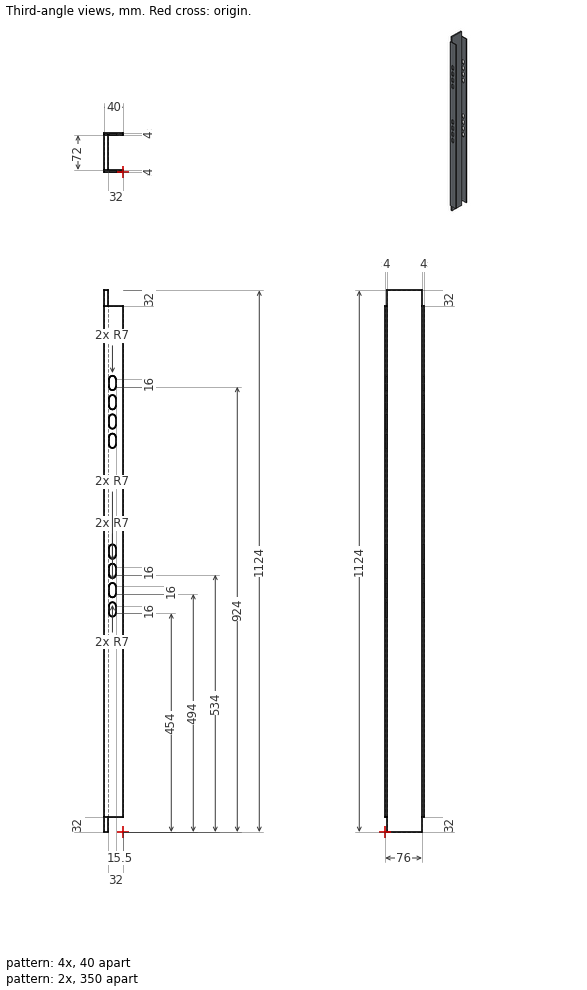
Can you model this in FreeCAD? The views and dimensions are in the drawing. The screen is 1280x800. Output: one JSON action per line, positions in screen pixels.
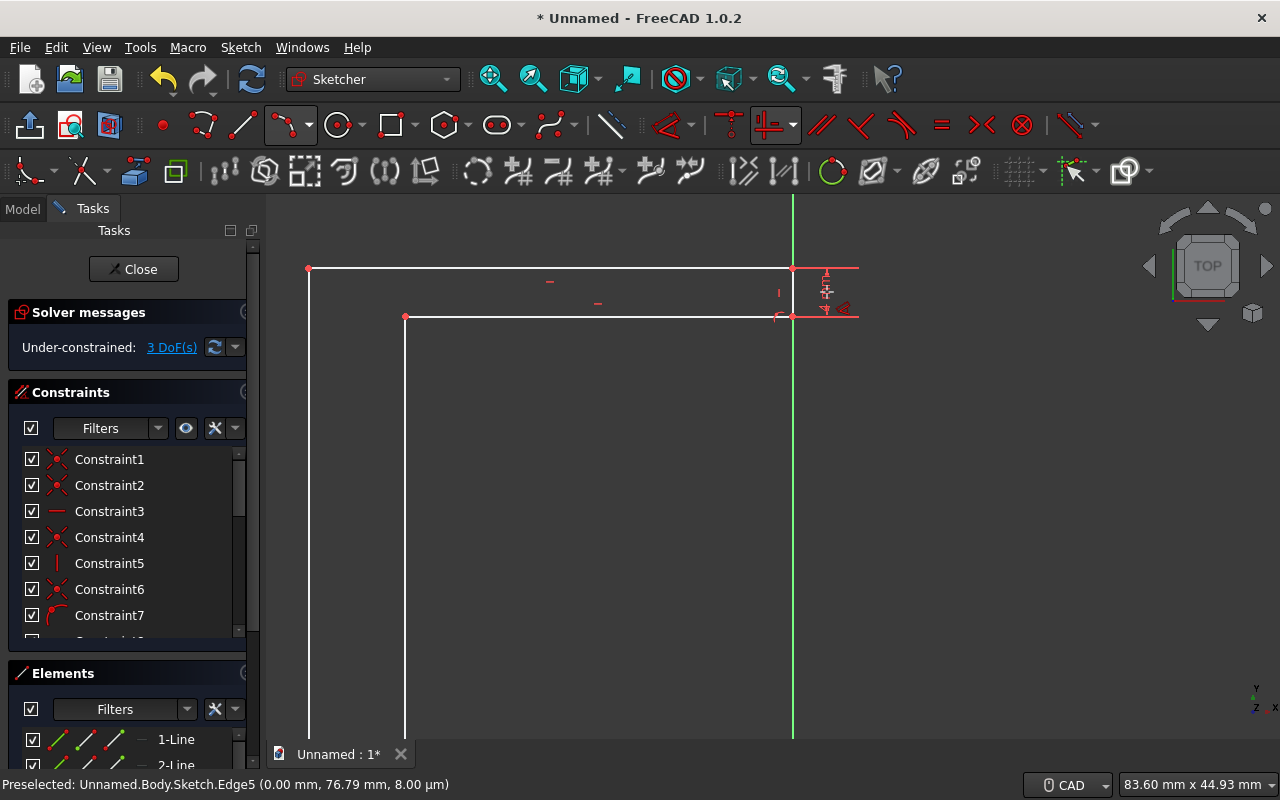
{"action": "scroll", "coordinate": [794, 302], "scroll_direction": "down", "scroll_amount": 5}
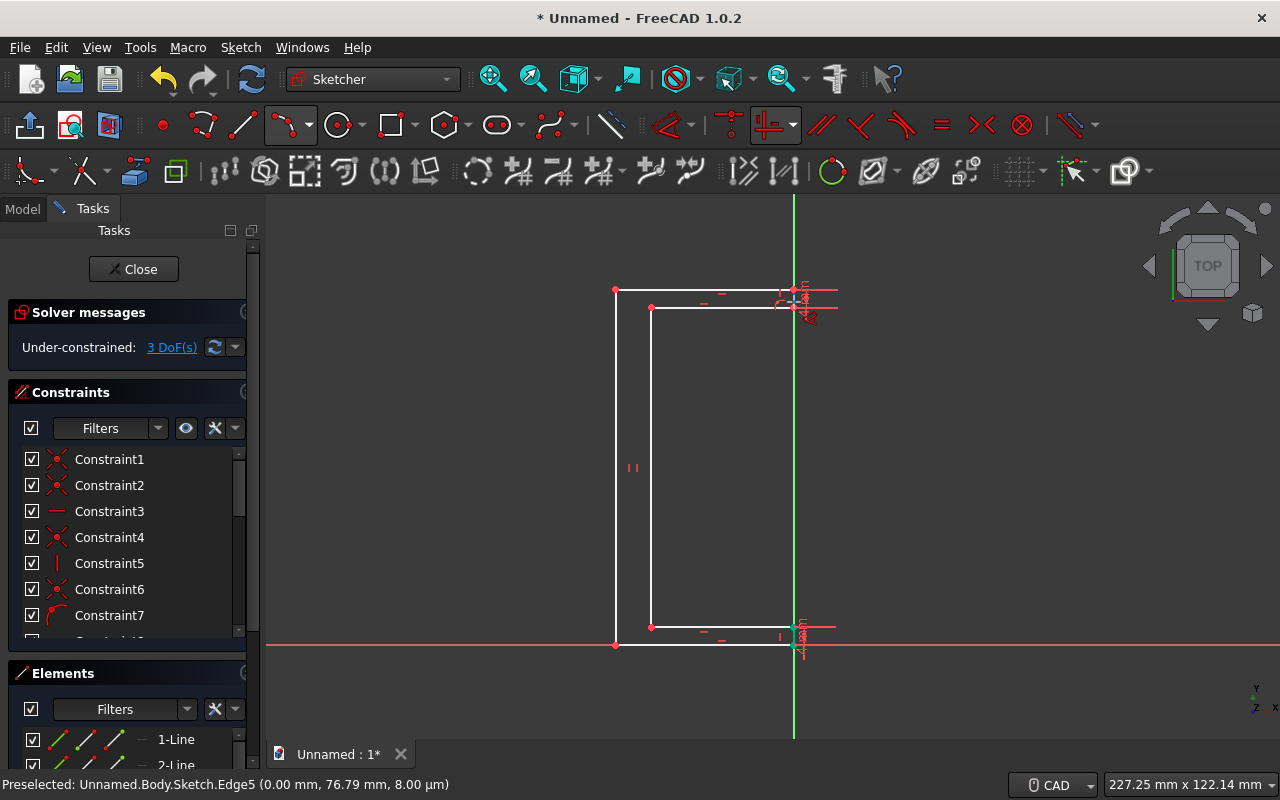
{"action": "left_click", "coordinate": [751, 627]}
{"action": "left_click", "coordinate": [723, 661]}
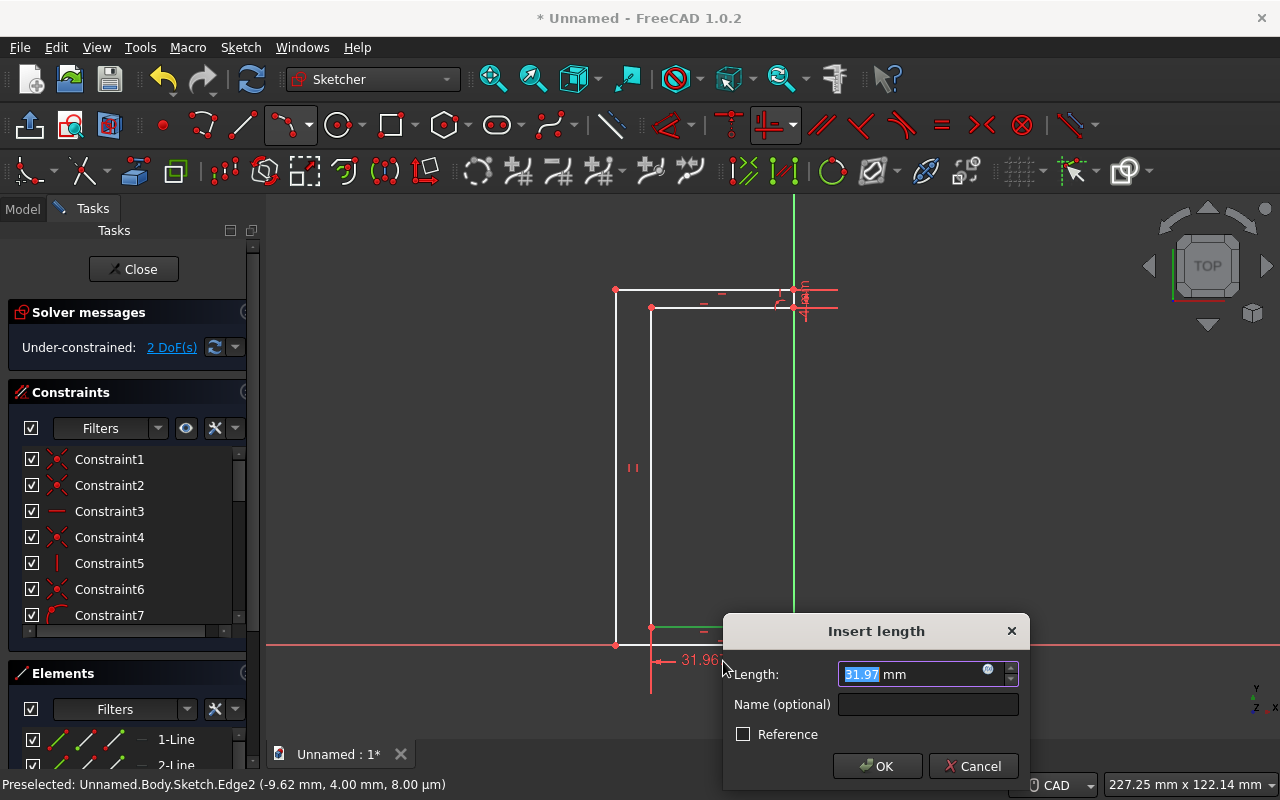
{"action": "type", "text": "32"}
{"action": "key", "text": "Return"}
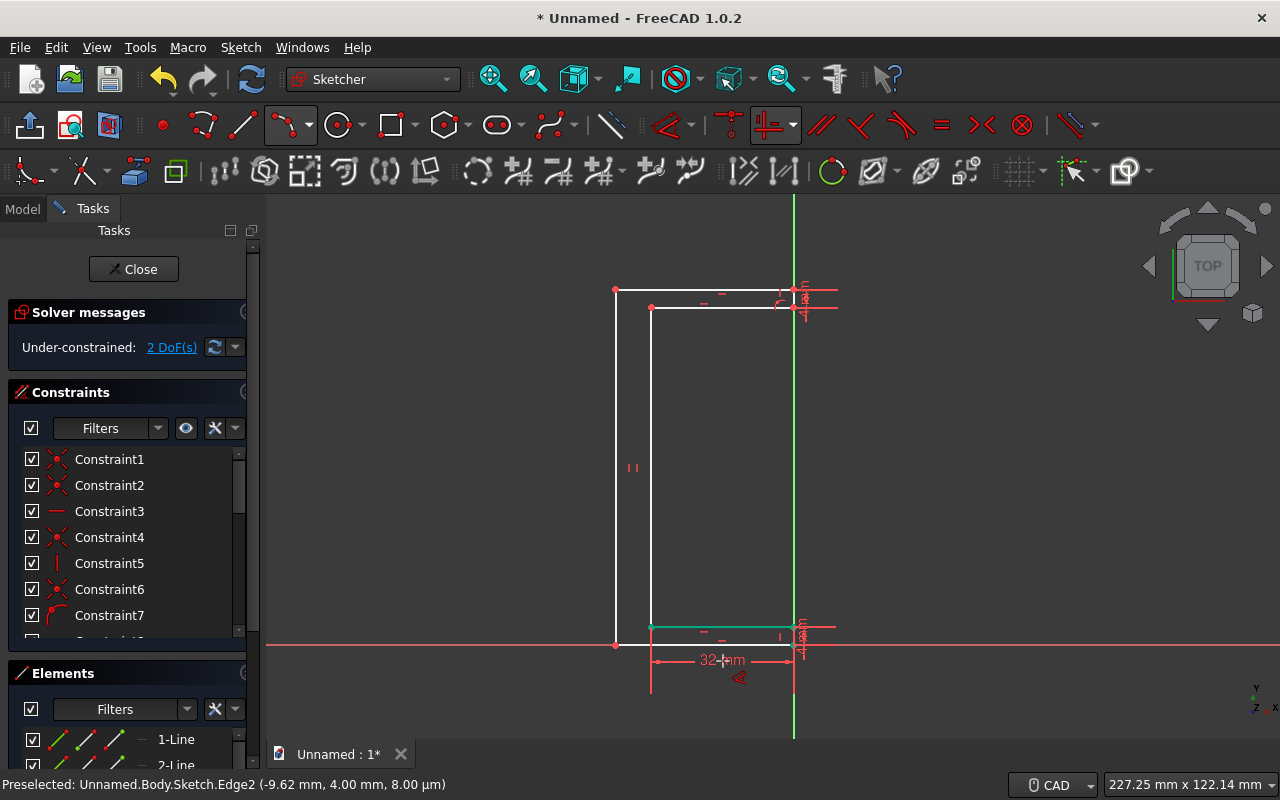
{"action": "left_click", "coordinate": [651, 531]}
{"action": "left_click", "coordinate": [685, 467]}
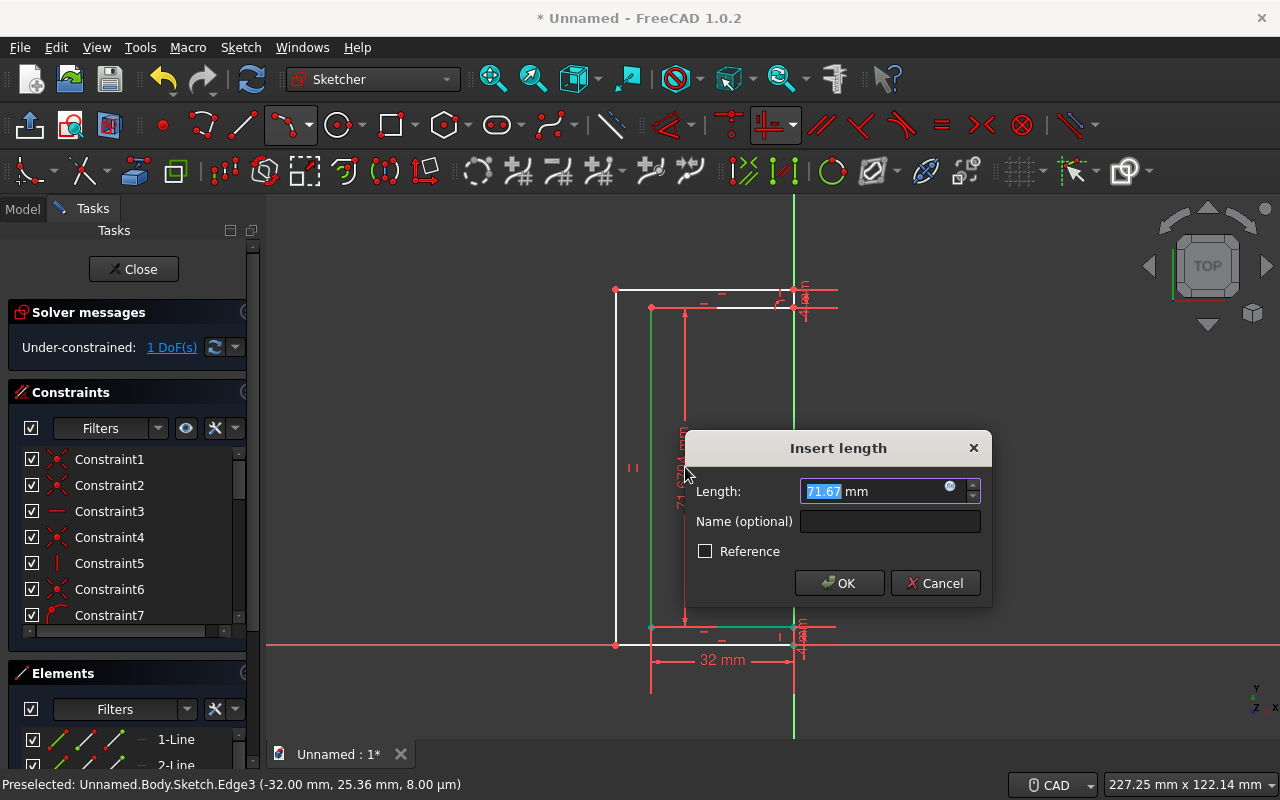
{"action": "type", "text": "72"}
{"action": "key", "text": "Return"}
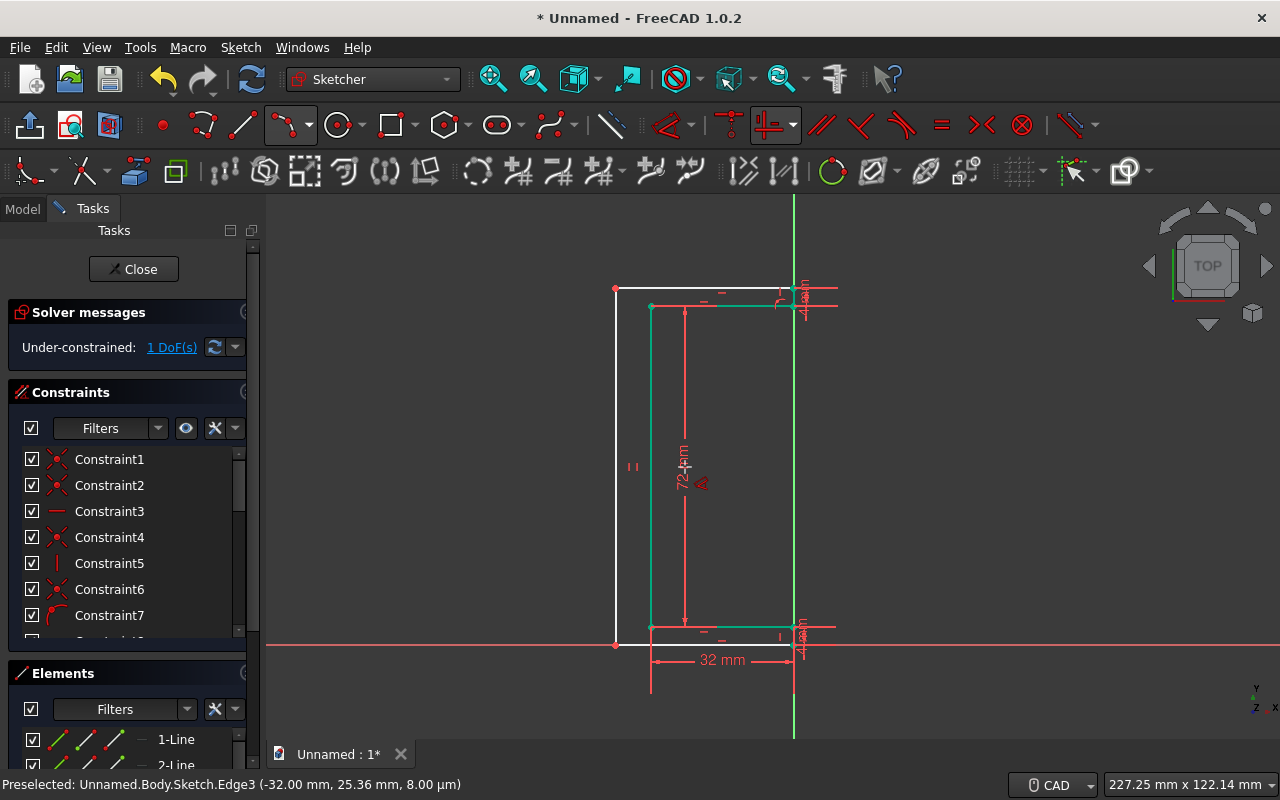
{"action": "left_click", "coordinate": [740, 288]}
{"action": "left_click", "coordinate": [705, 254]}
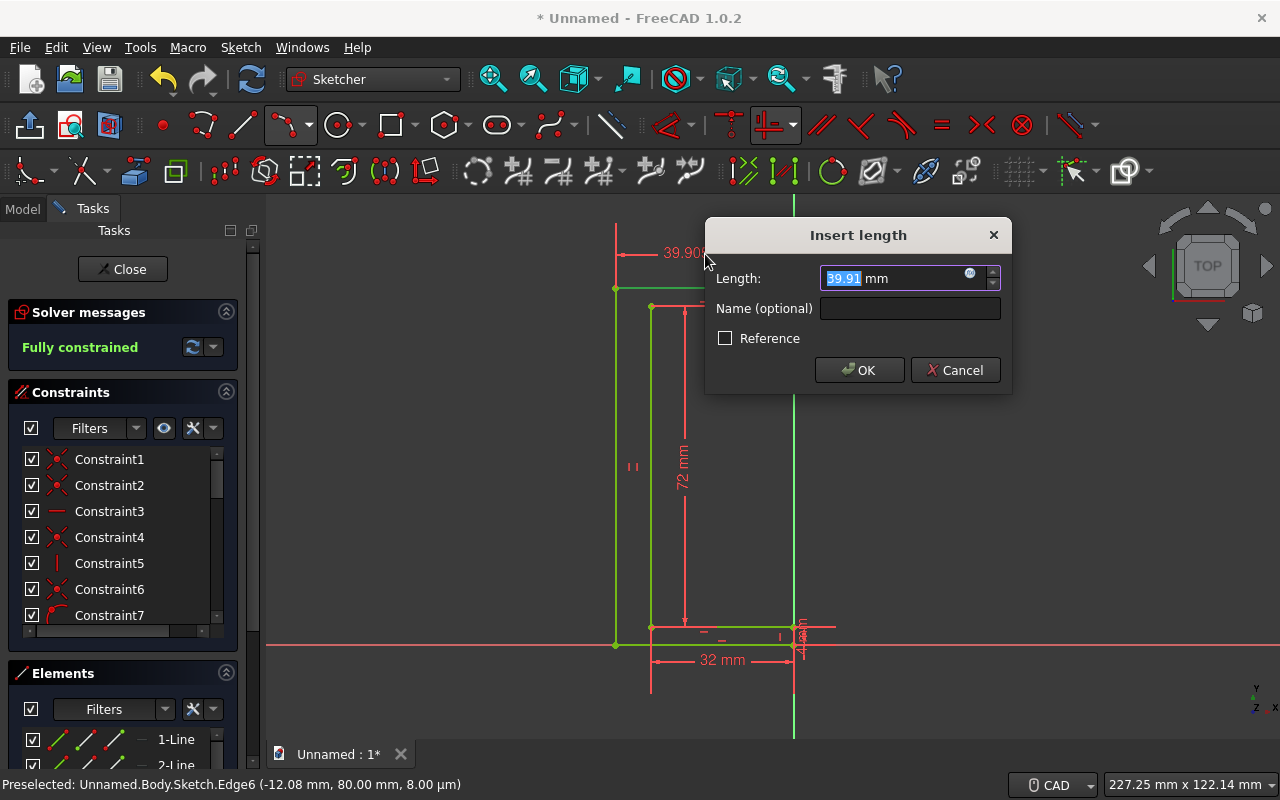
{"action": "type", "text": "40"}
{"action": "key", "text": "Return"}
{"action": "key", "text": "Escape"}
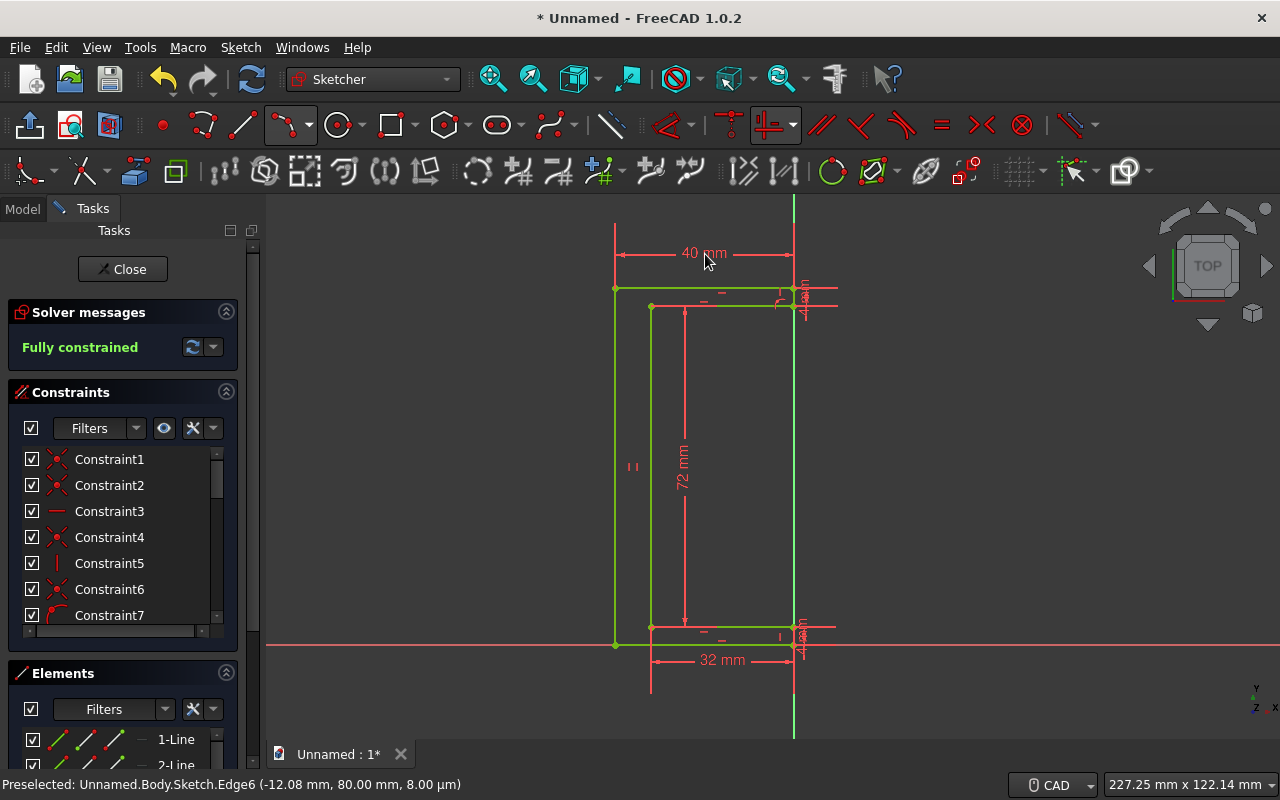
{"action": "left_click", "coordinate": [123, 269]}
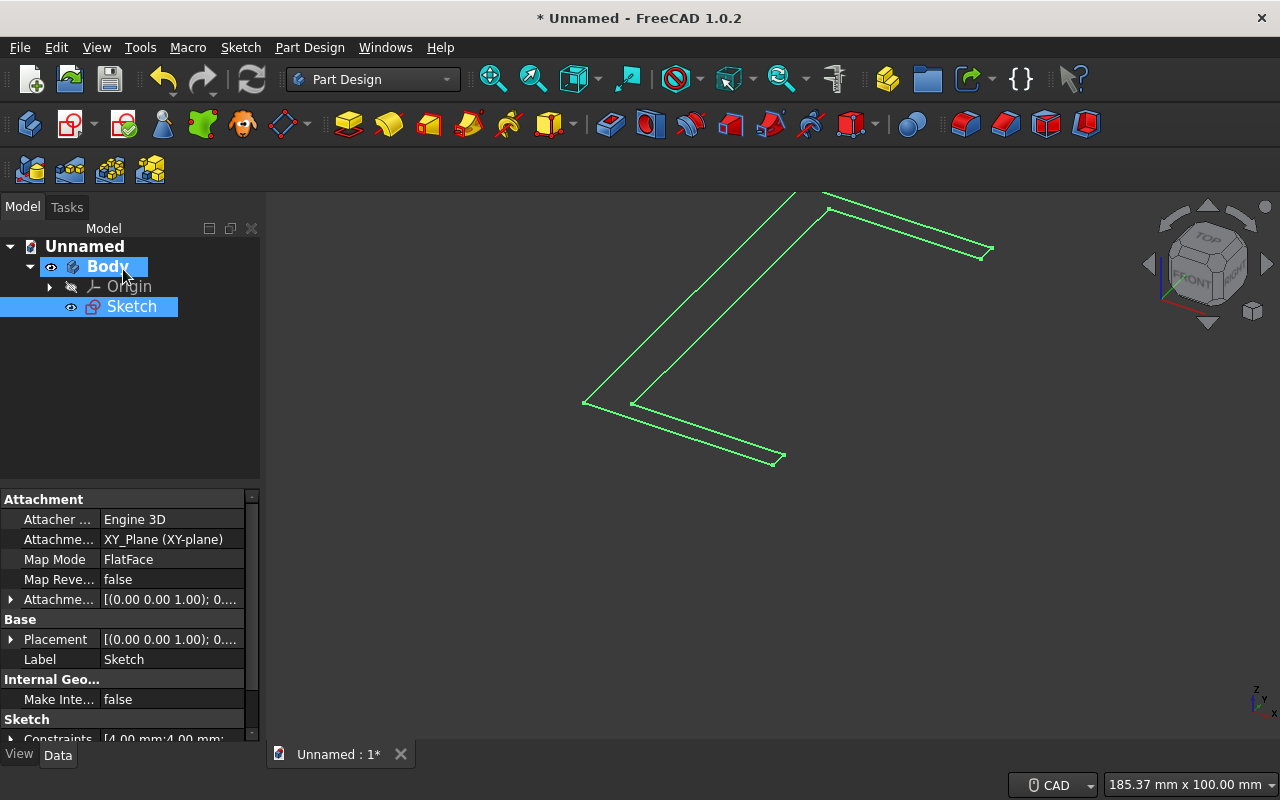
{"action": "left_click", "coordinate": [350, 124]}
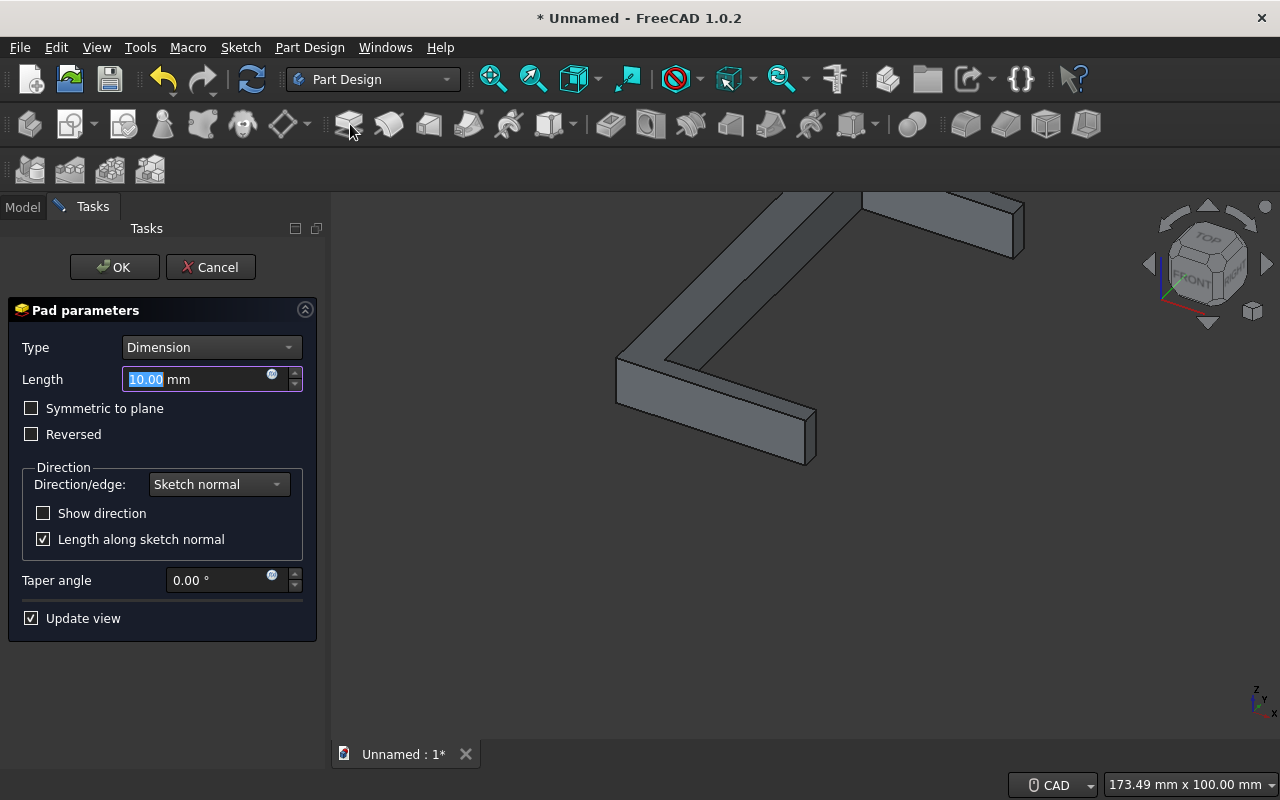
{"action": "type", "text": "1124"}
{"action": "key", "text": "Tab"}